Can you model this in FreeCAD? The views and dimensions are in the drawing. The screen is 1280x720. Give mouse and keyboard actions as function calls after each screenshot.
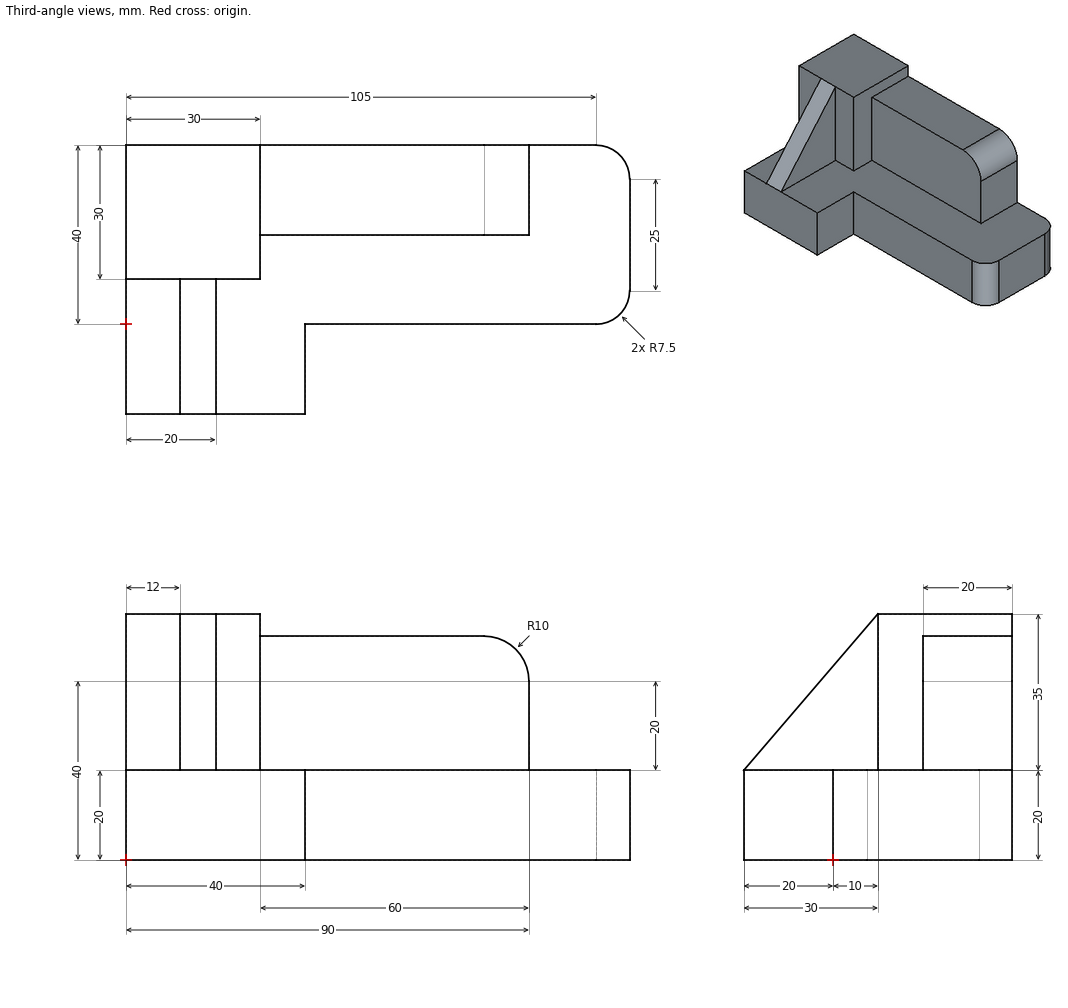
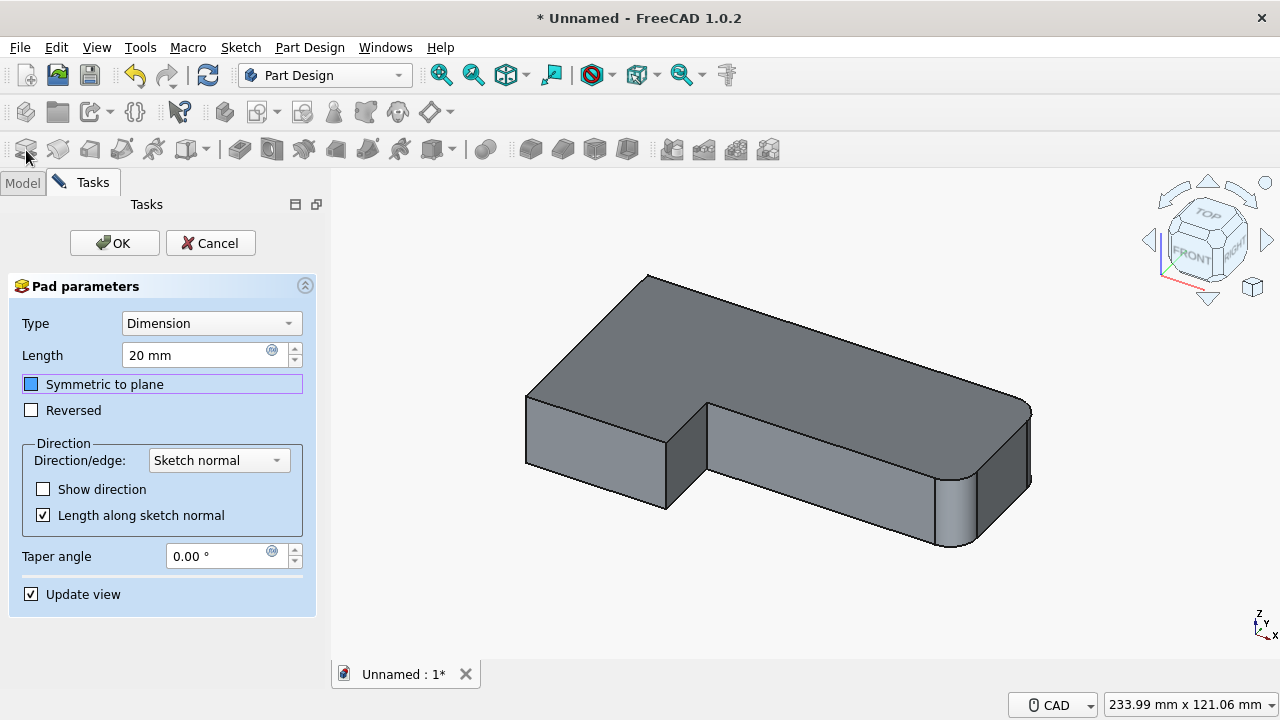
click(115, 243)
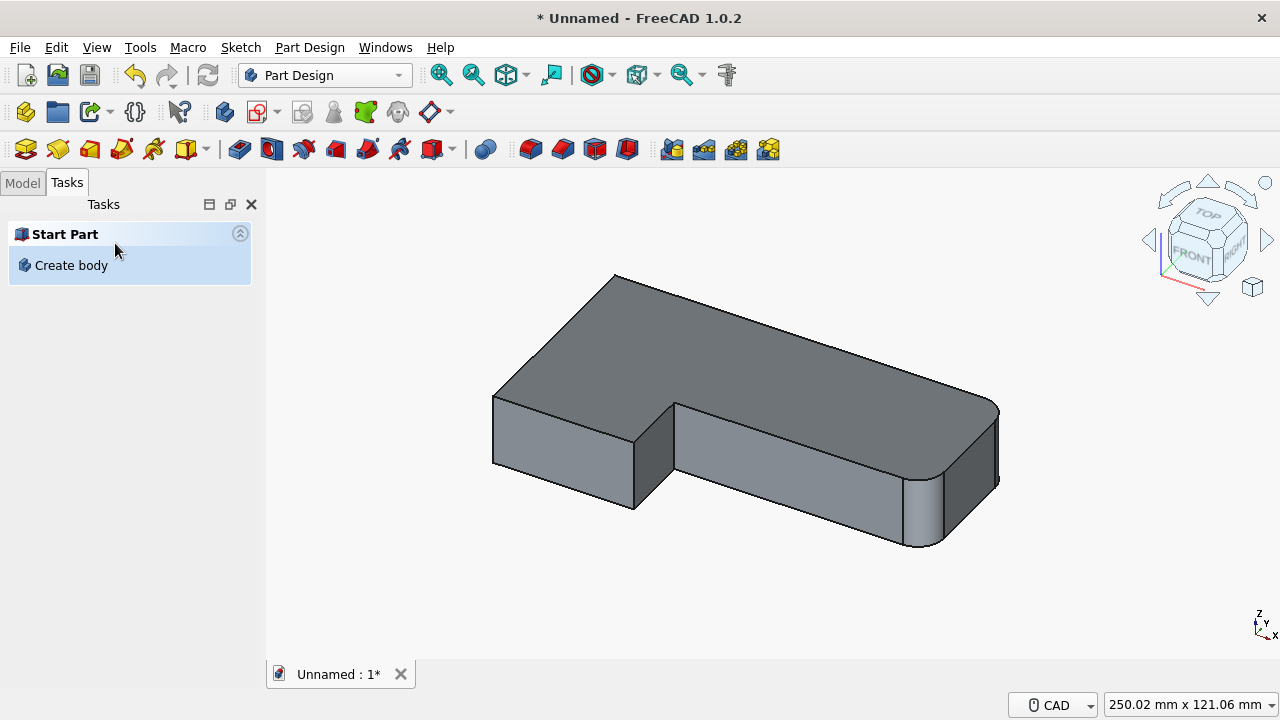
click(656, 346)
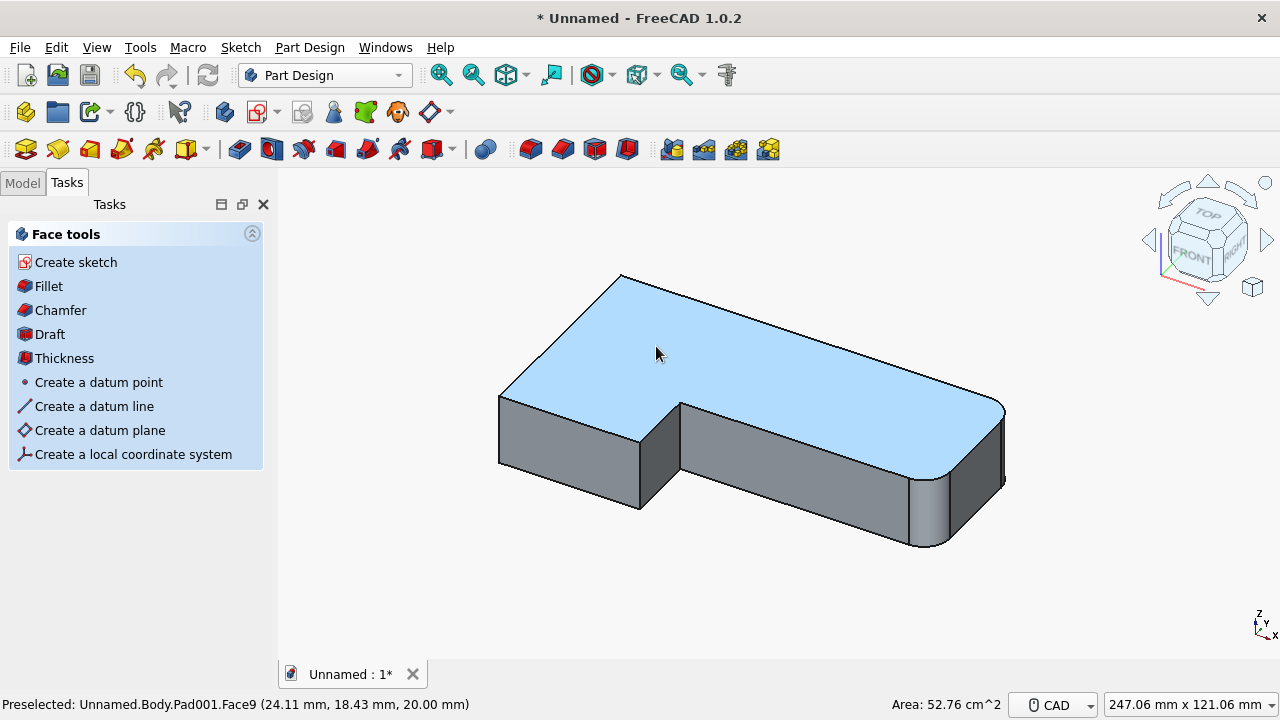
click(258, 112)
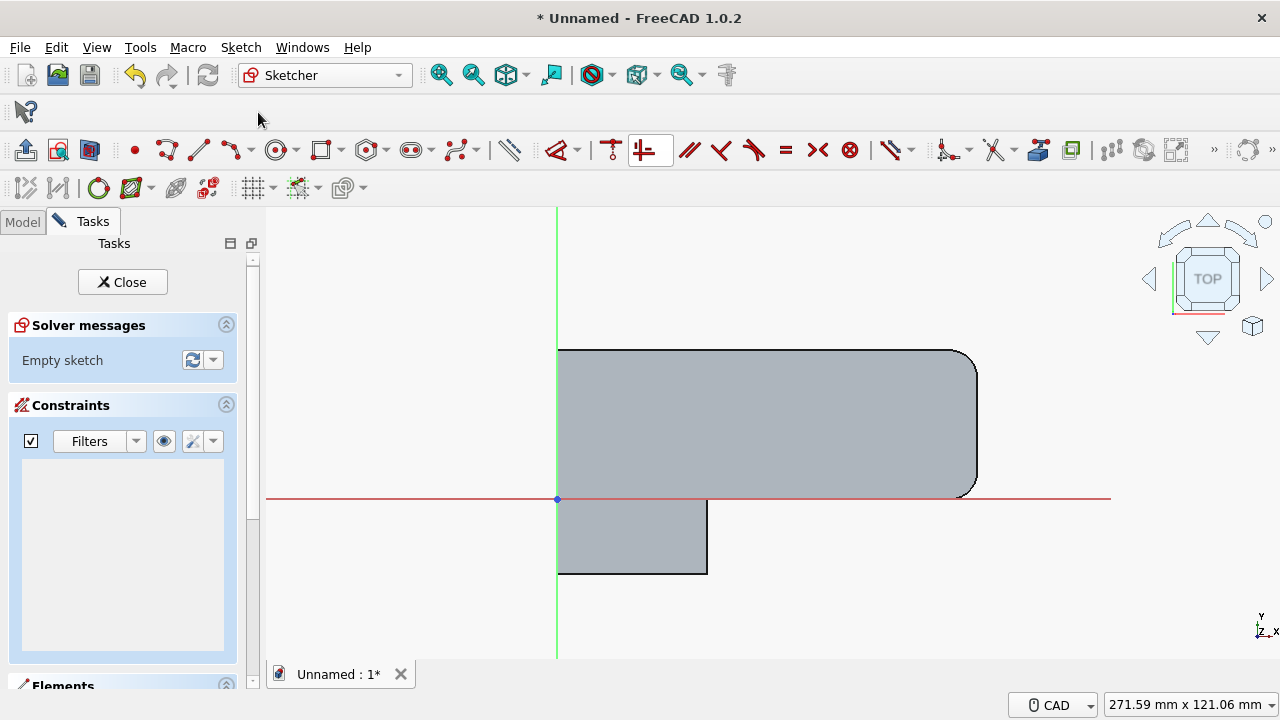
scroll(502, 415, up, 3)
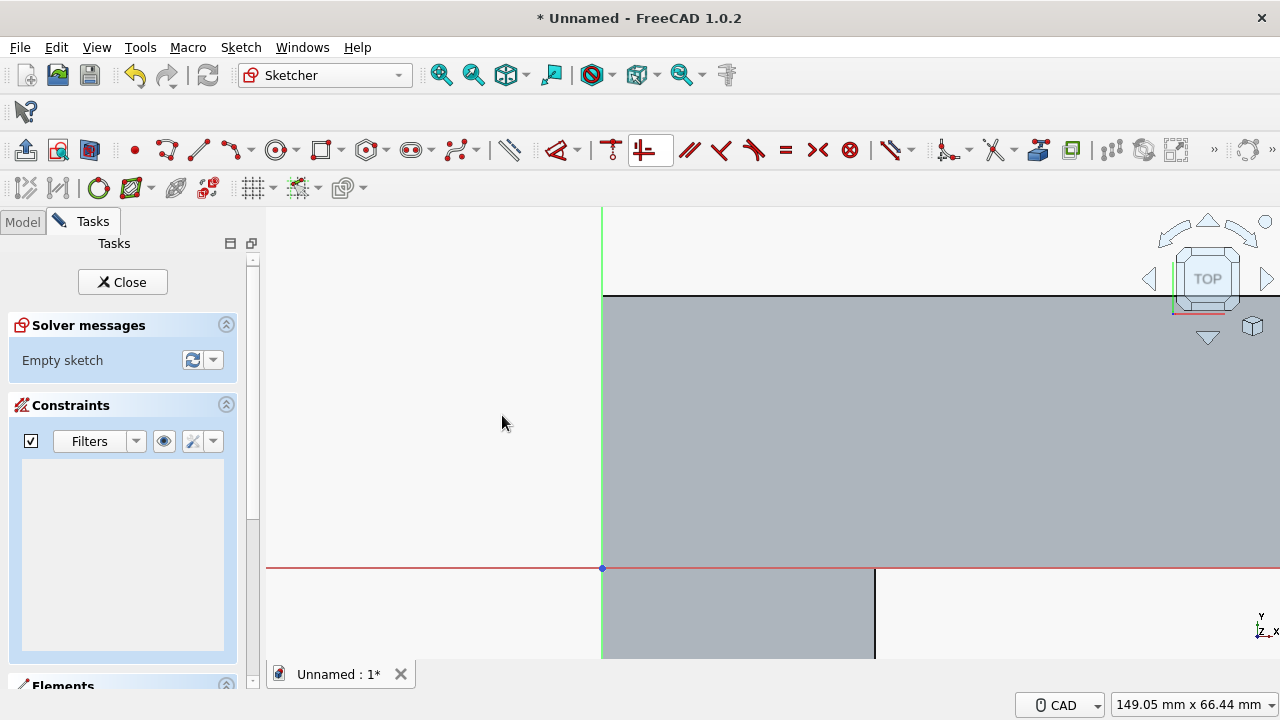
key(g)
key(r)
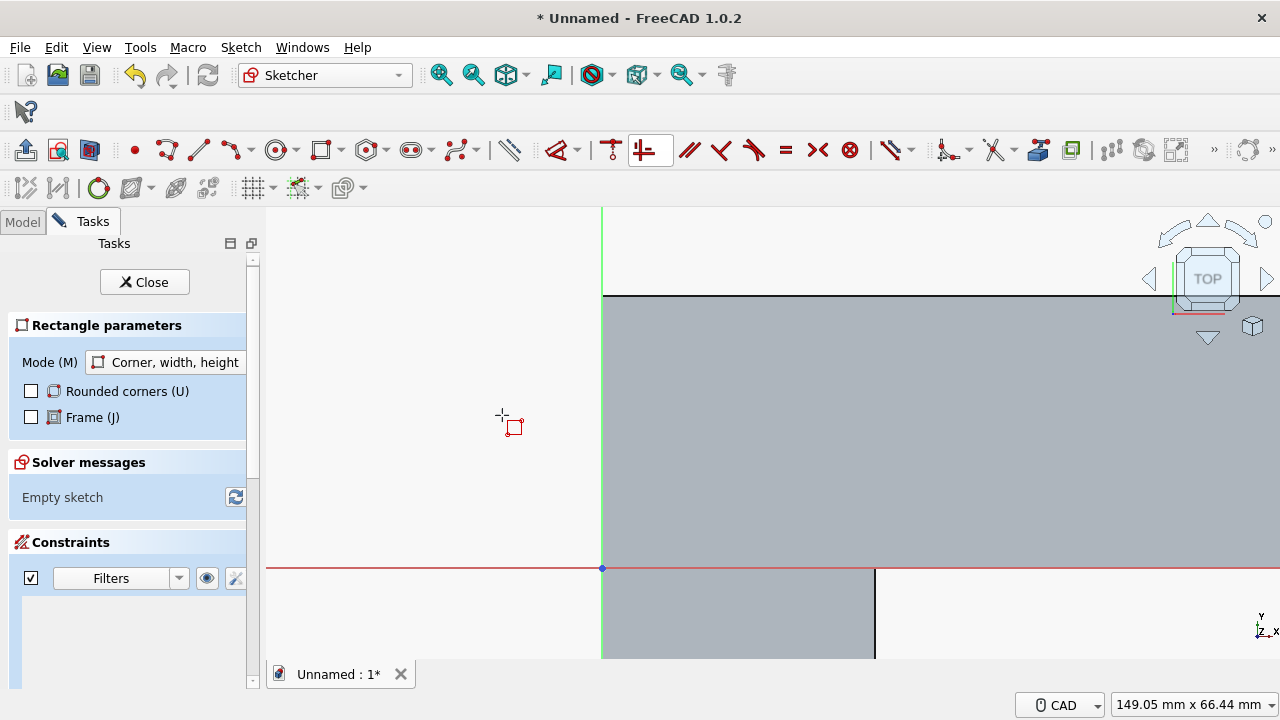
click(602, 296)
move(807, 500)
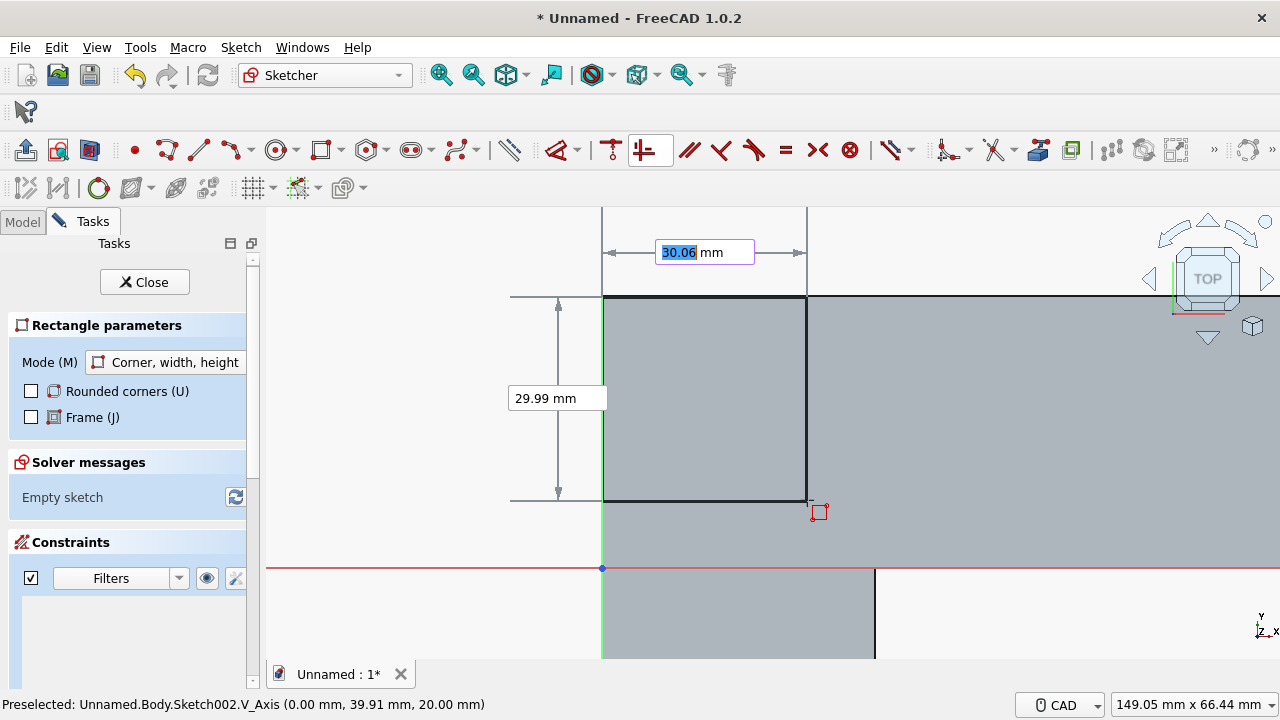
text(30)
key(Tab)
text(30)
key(Return)
key(Escape)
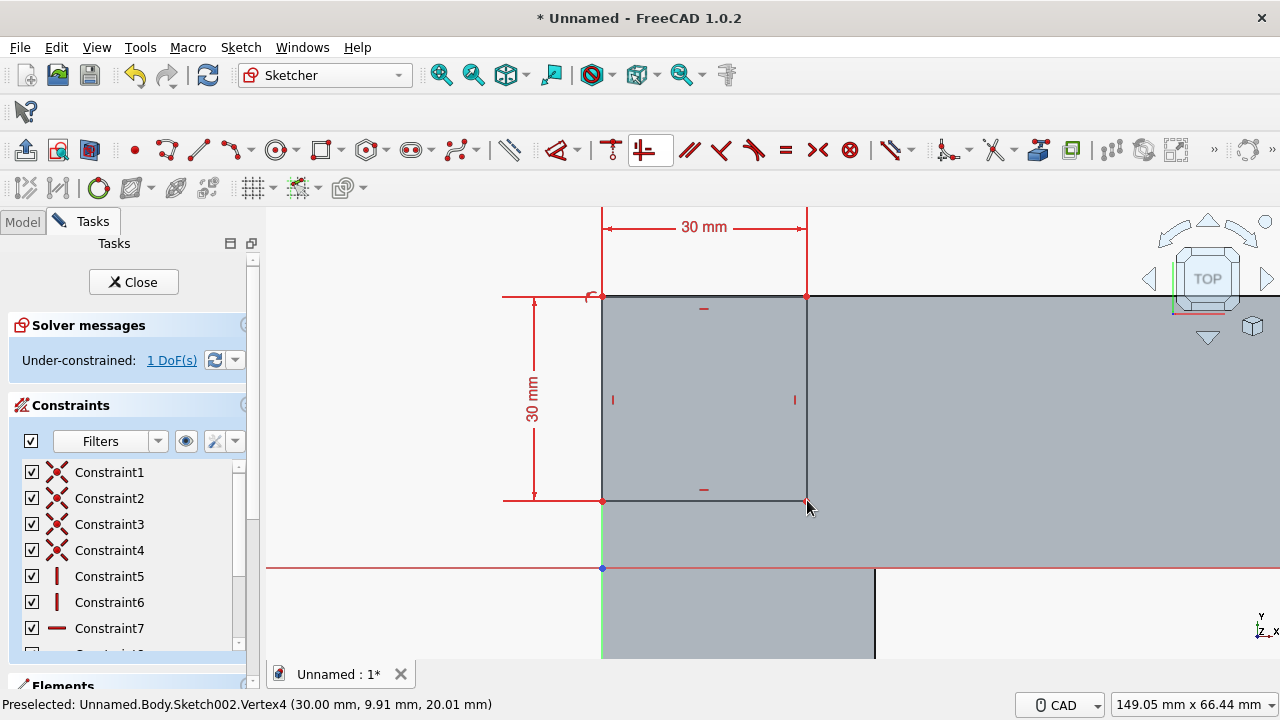
key(d)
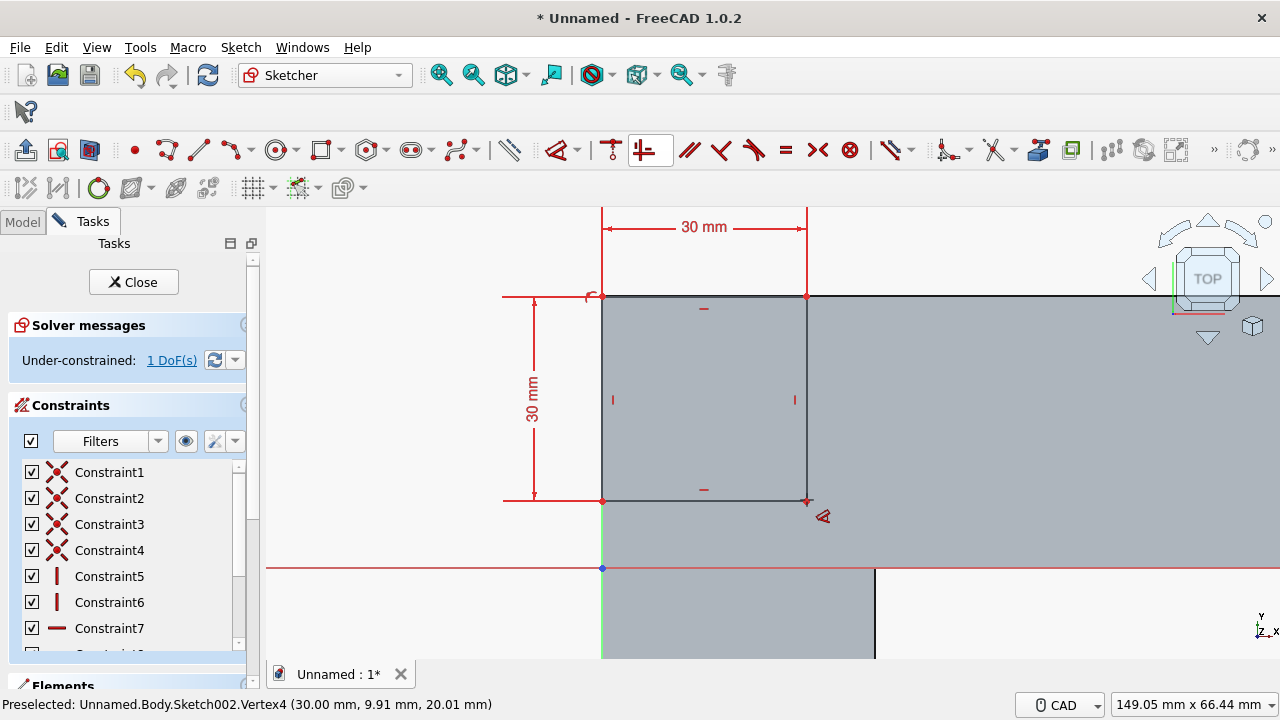
click(602, 297)
click(568, 433)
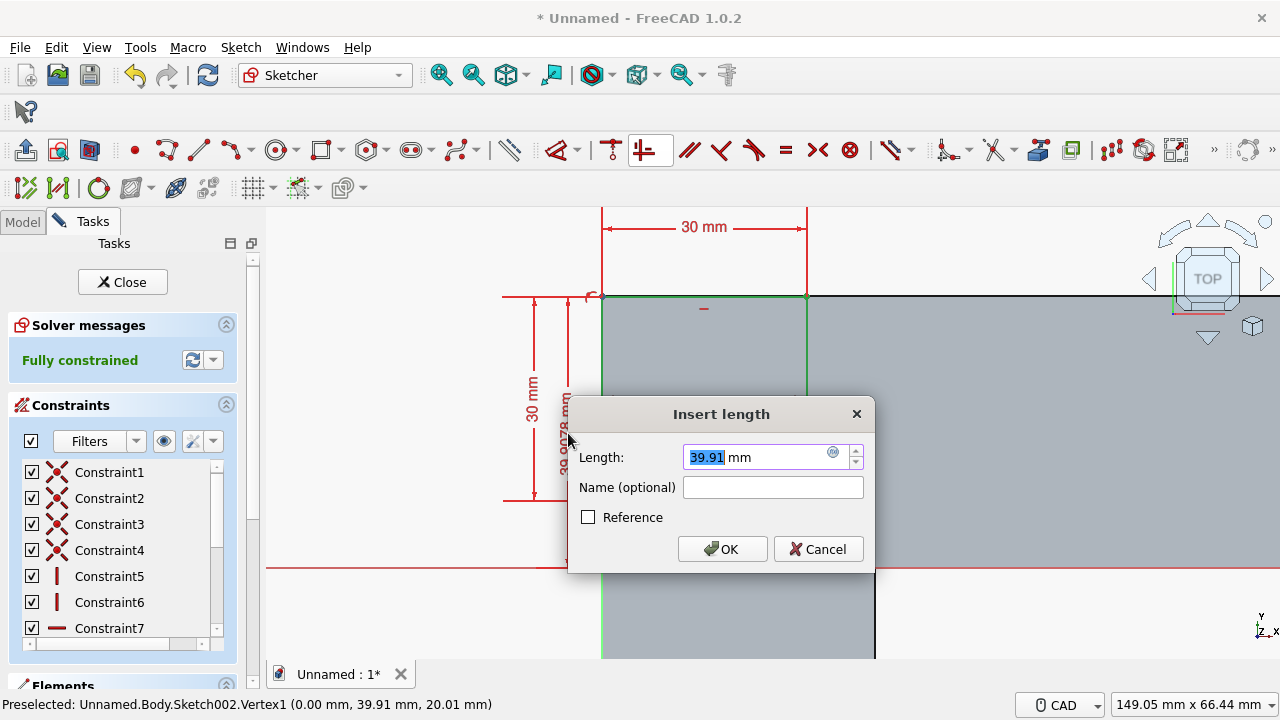
text(40)
key(Return)
key(Escape)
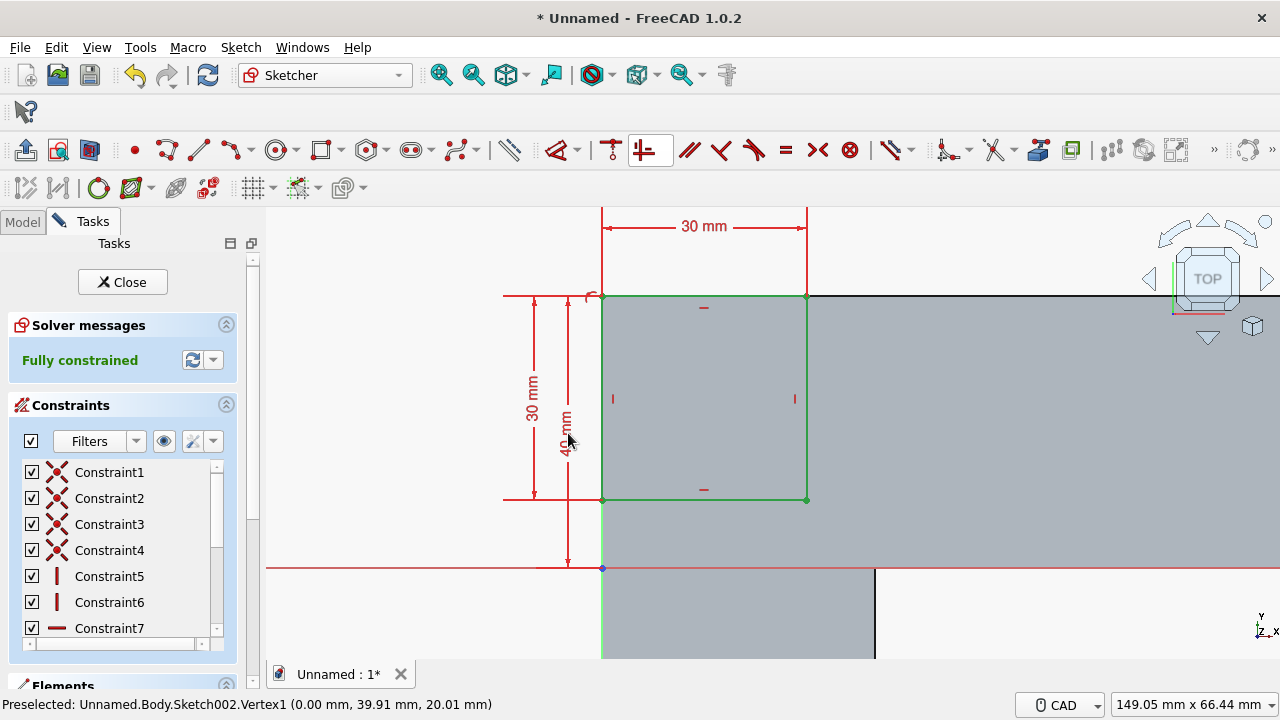
click(123, 282)